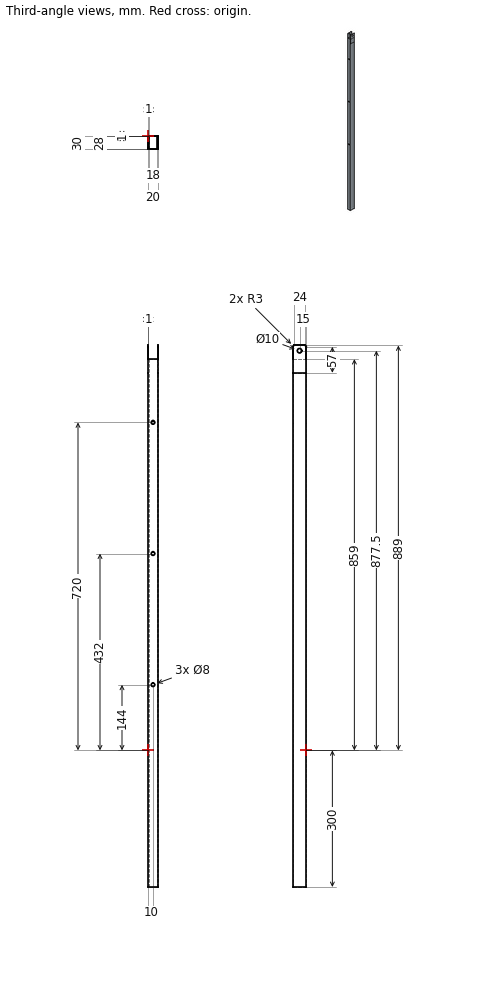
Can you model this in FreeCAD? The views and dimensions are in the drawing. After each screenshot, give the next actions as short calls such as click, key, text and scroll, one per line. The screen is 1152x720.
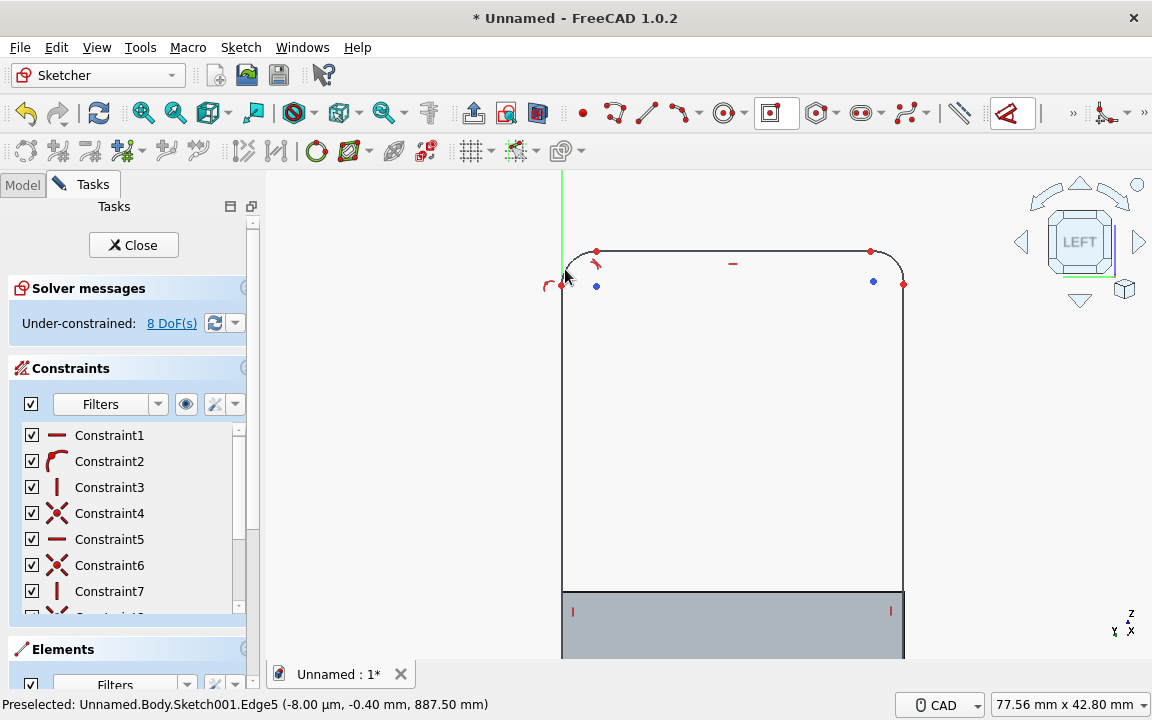
click(789, 251)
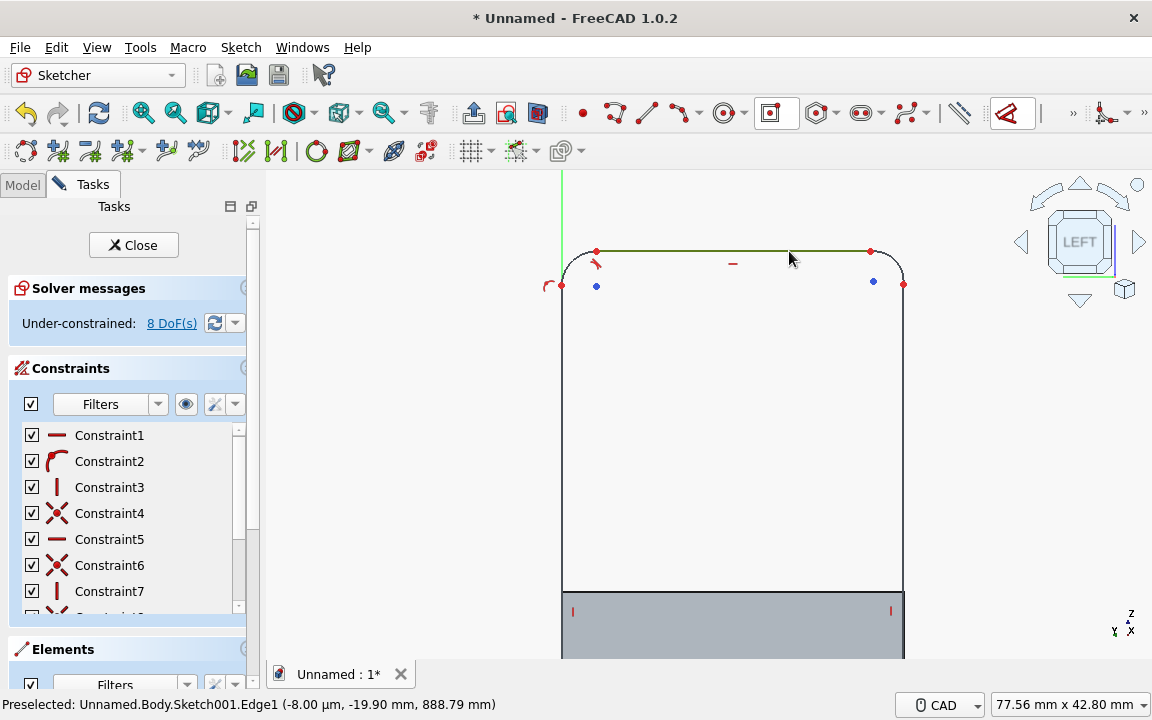
click(901, 269)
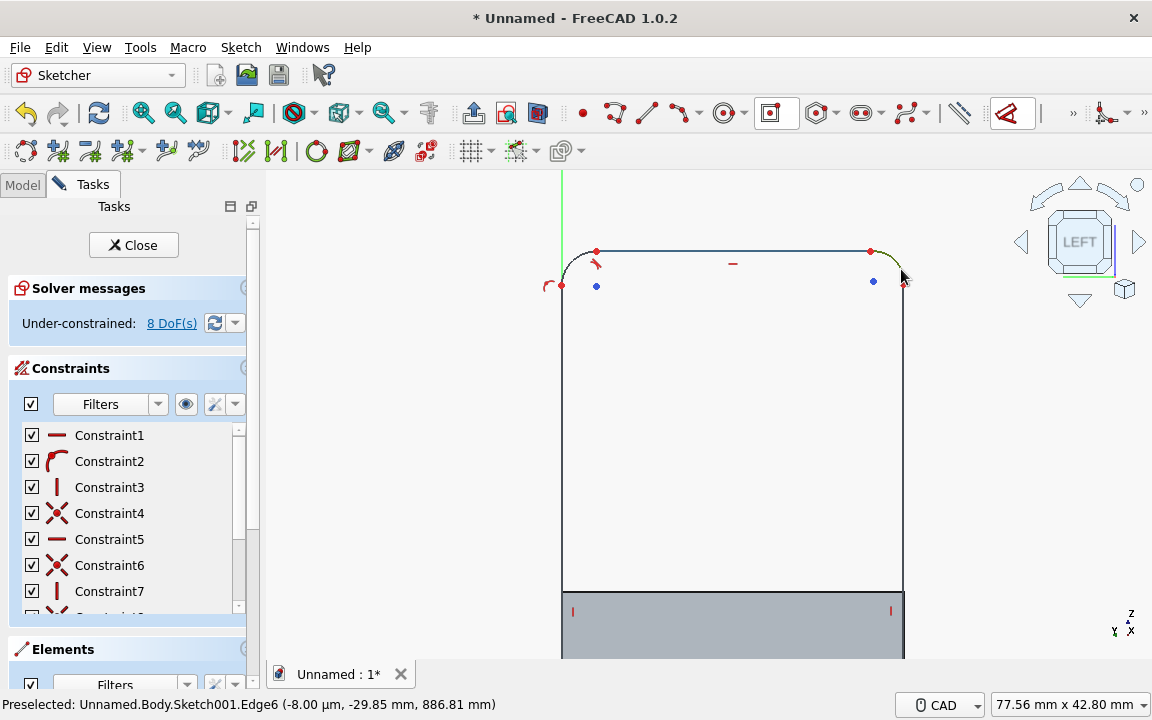
key(t)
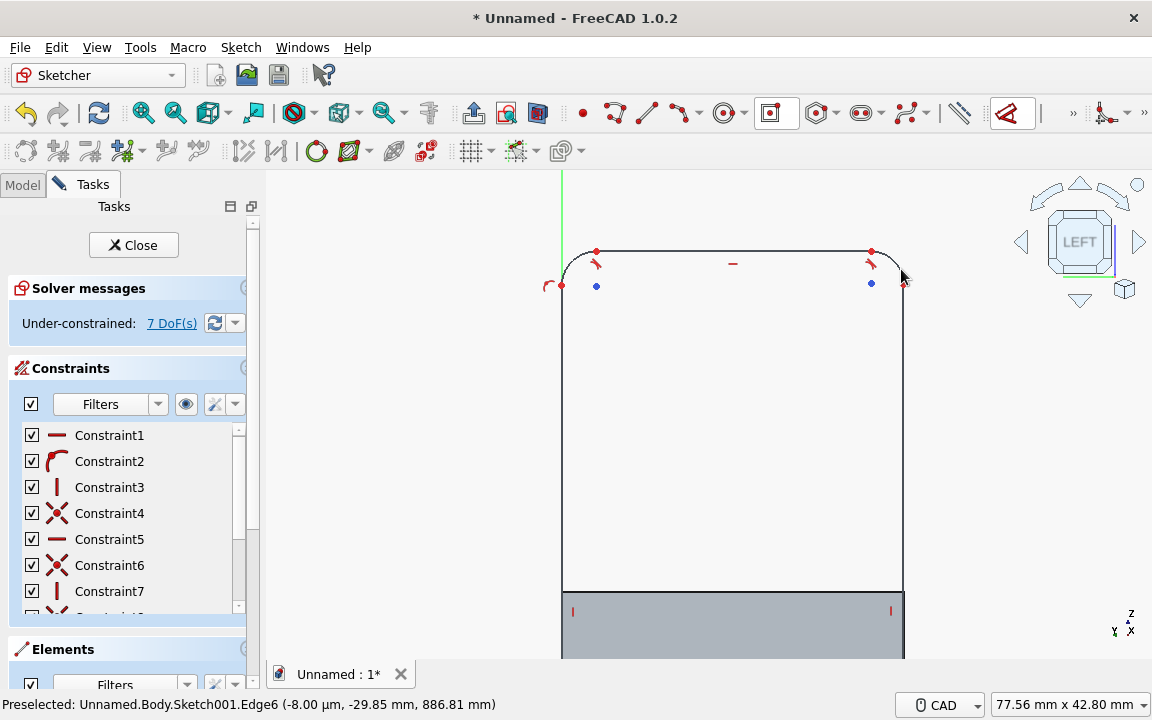
click(562, 481)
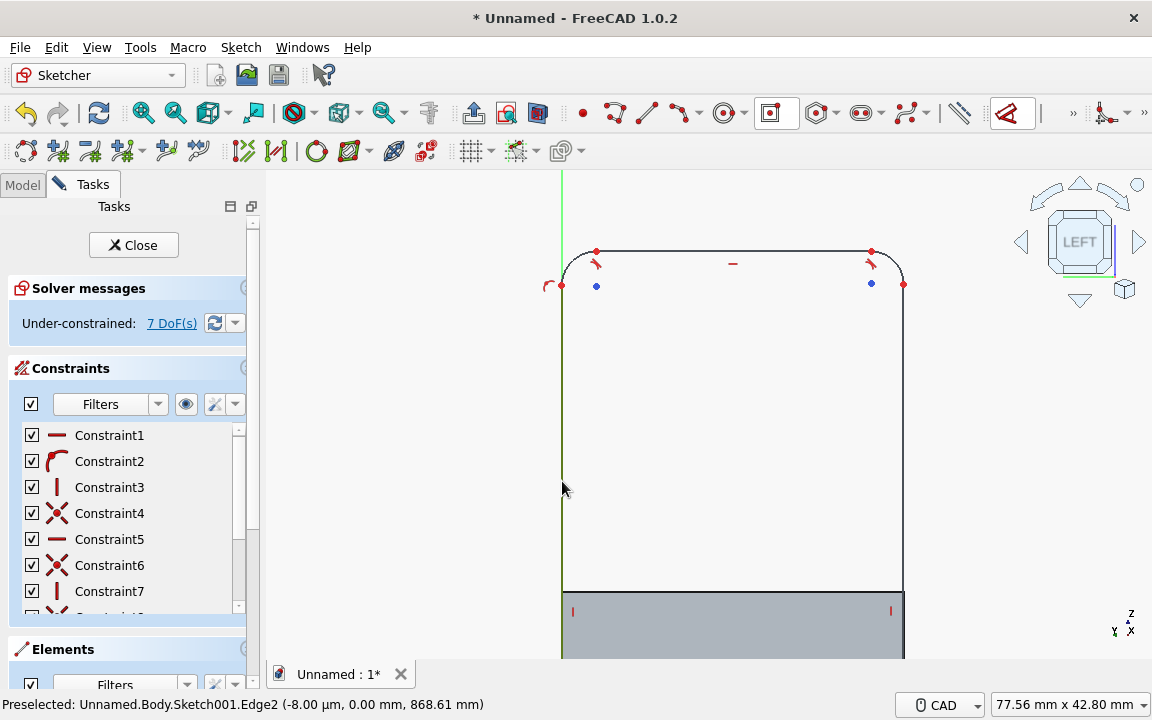
click(581, 255)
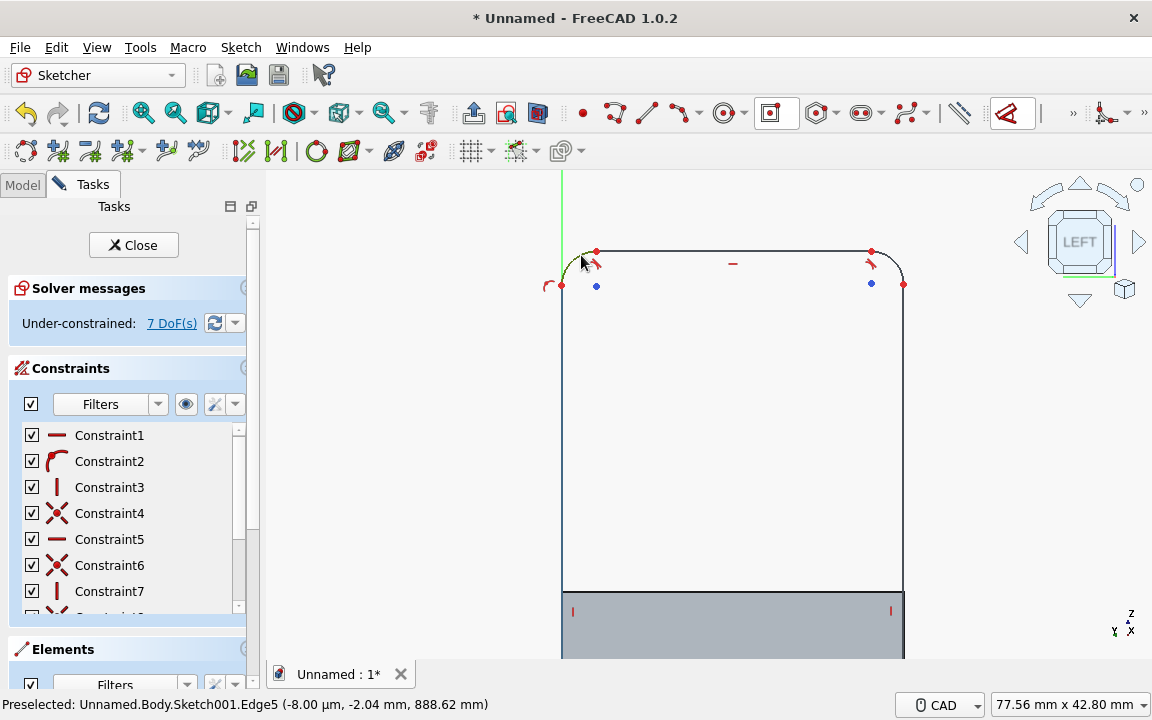
key(t)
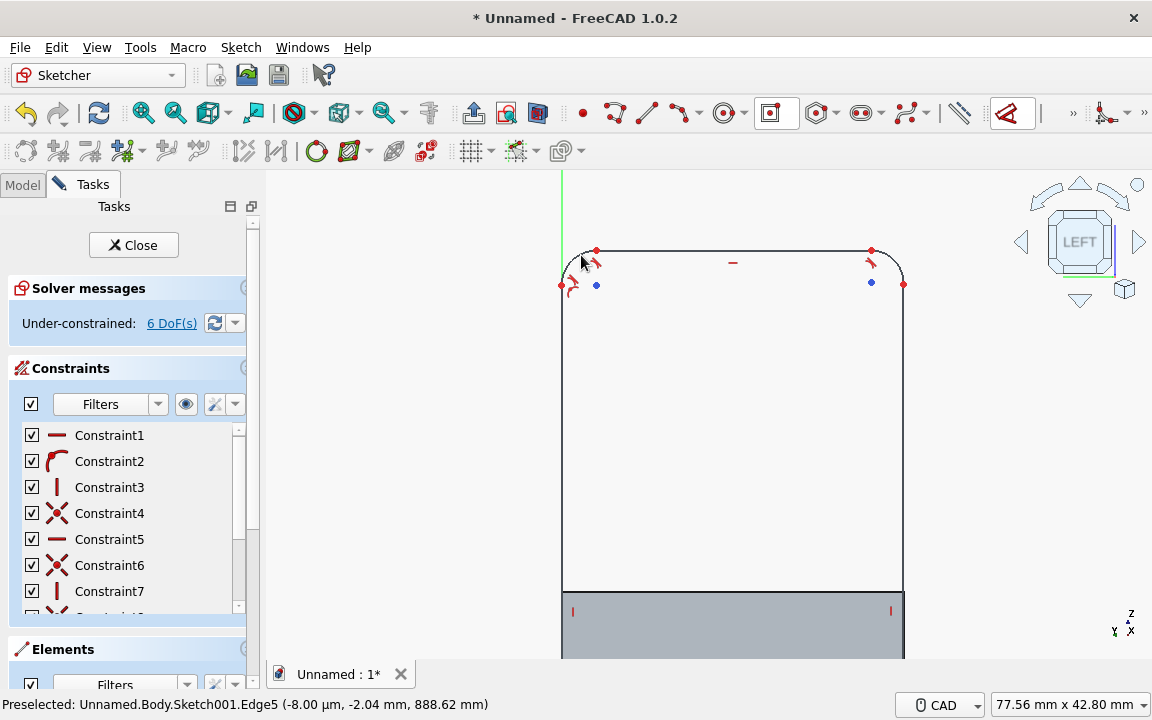
click(903, 480)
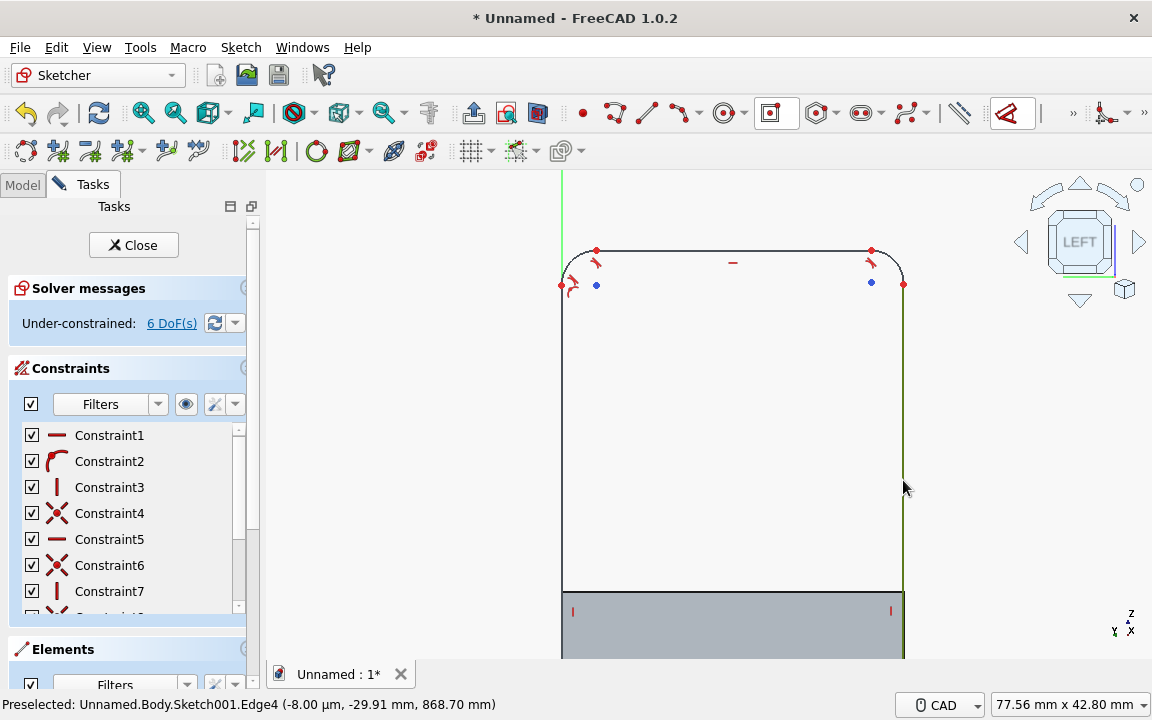
click(900, 269)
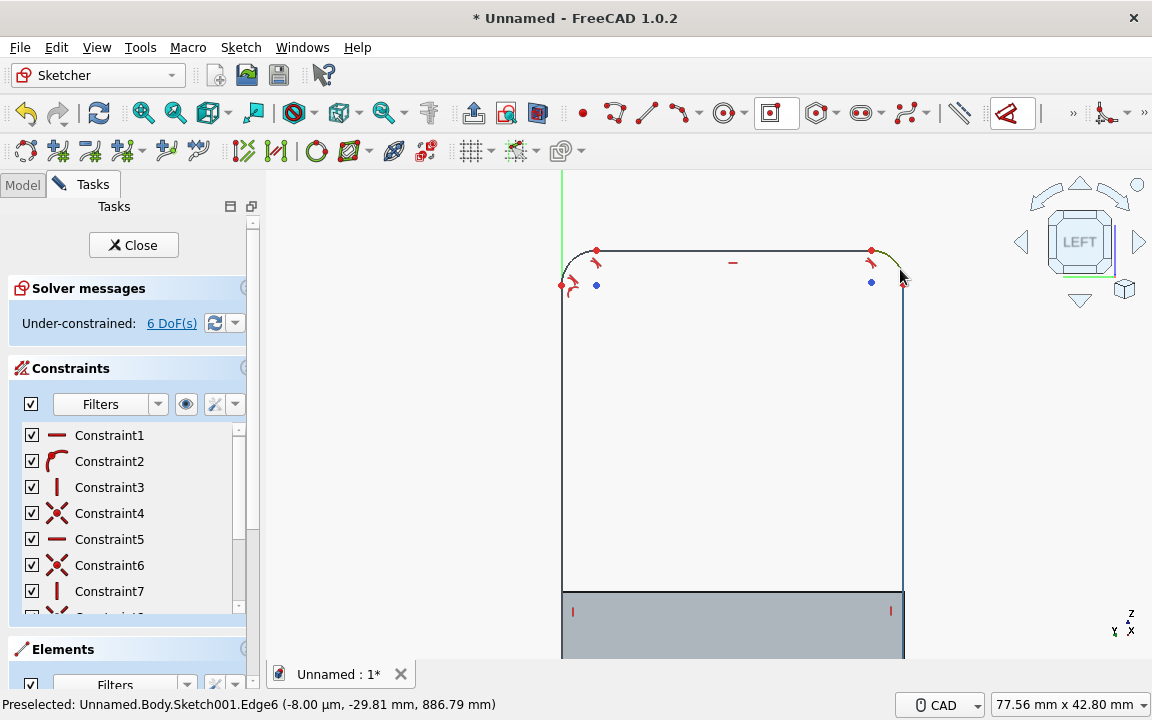
key(t)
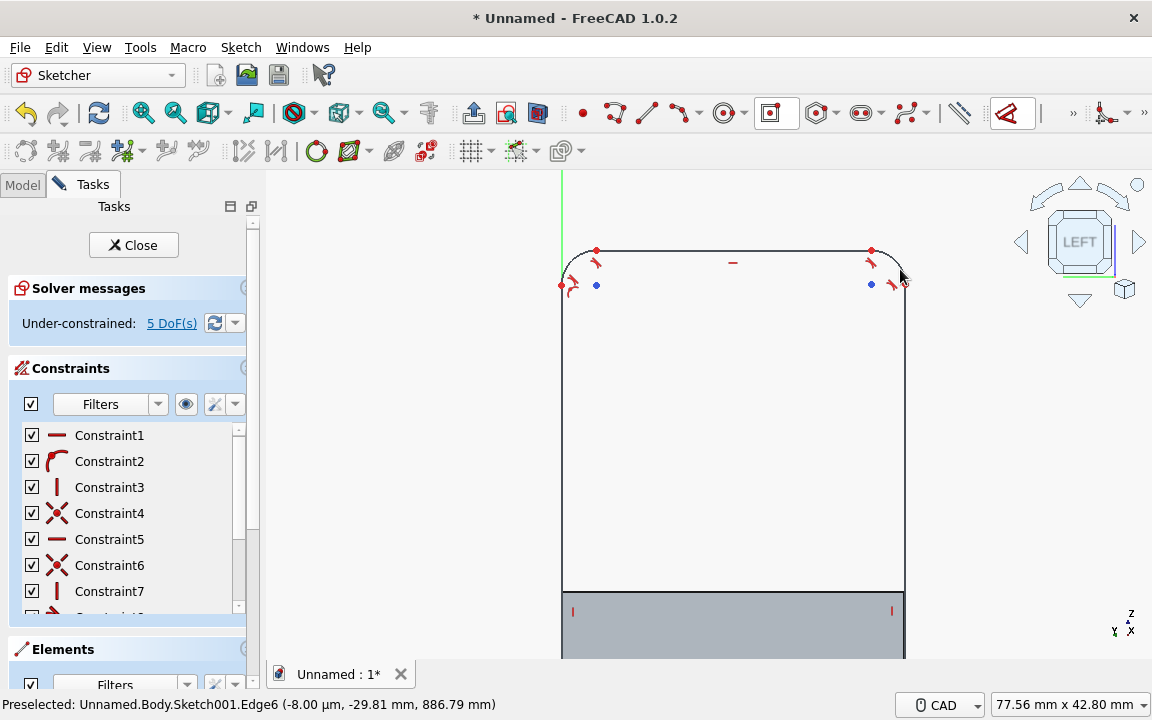
click(581, 254)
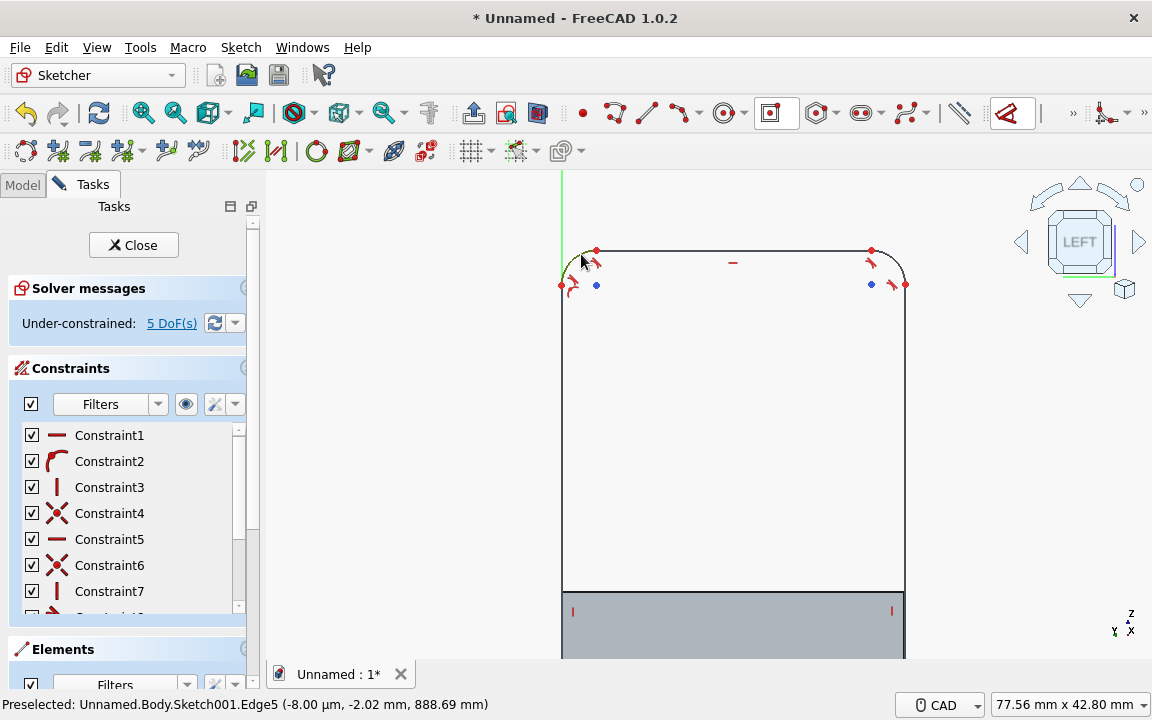
click(901, 269)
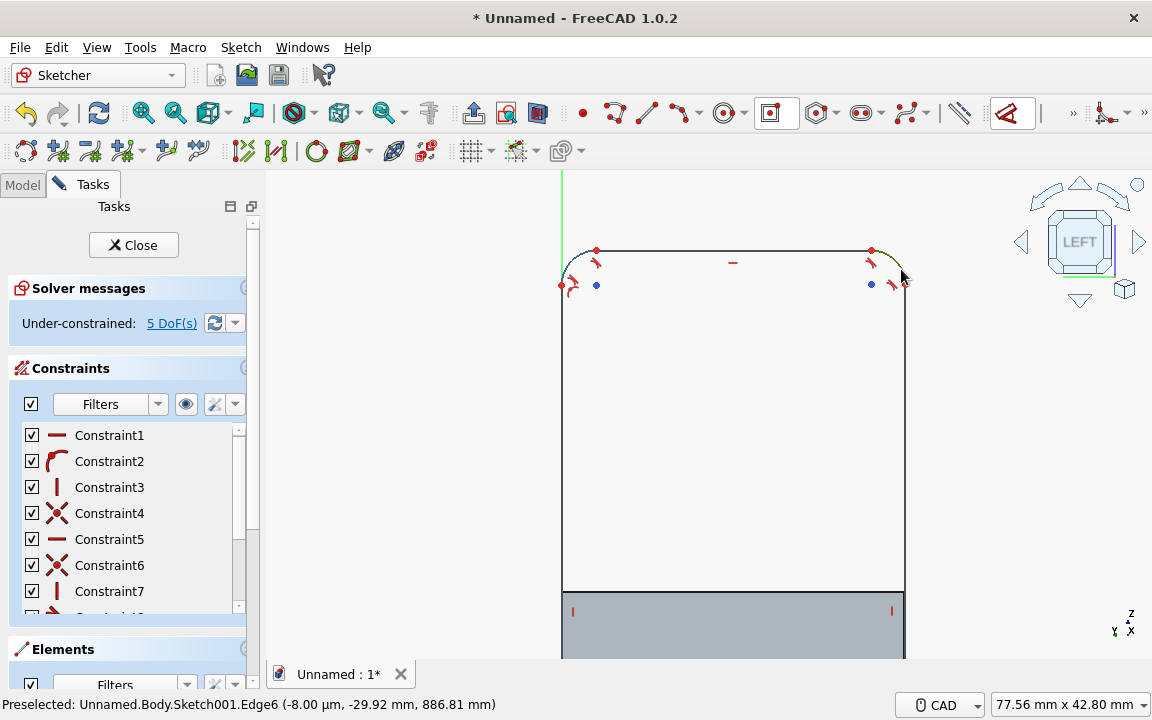
key(e)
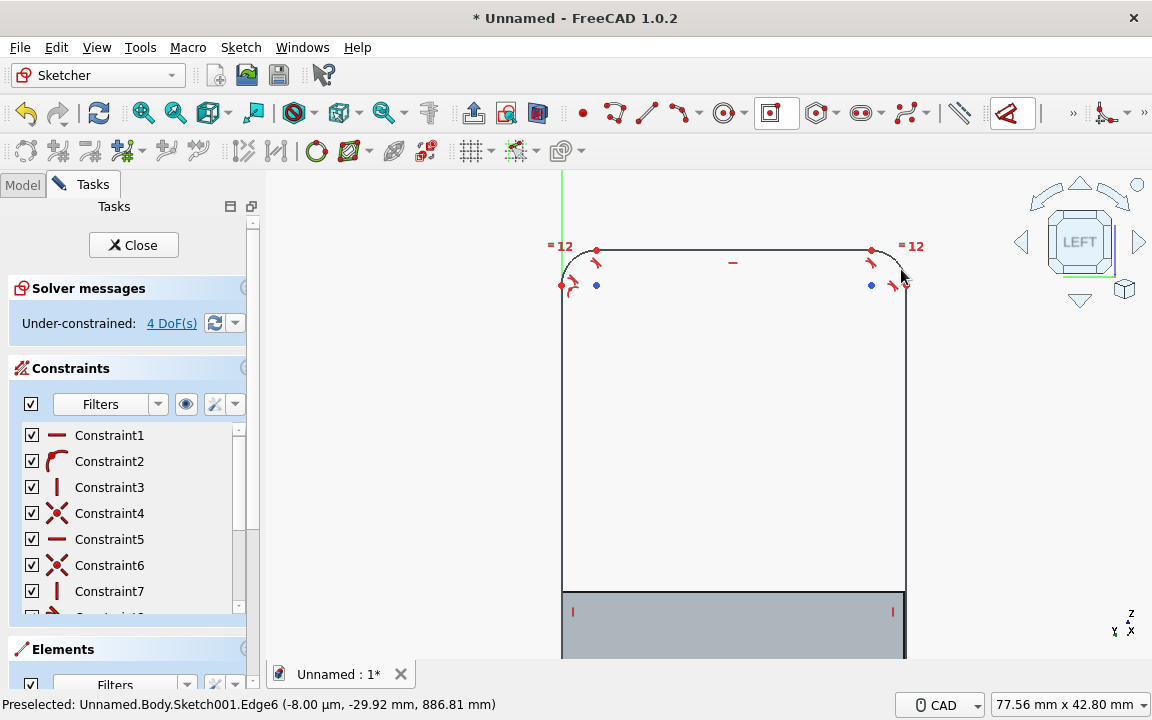
click(581, 254)